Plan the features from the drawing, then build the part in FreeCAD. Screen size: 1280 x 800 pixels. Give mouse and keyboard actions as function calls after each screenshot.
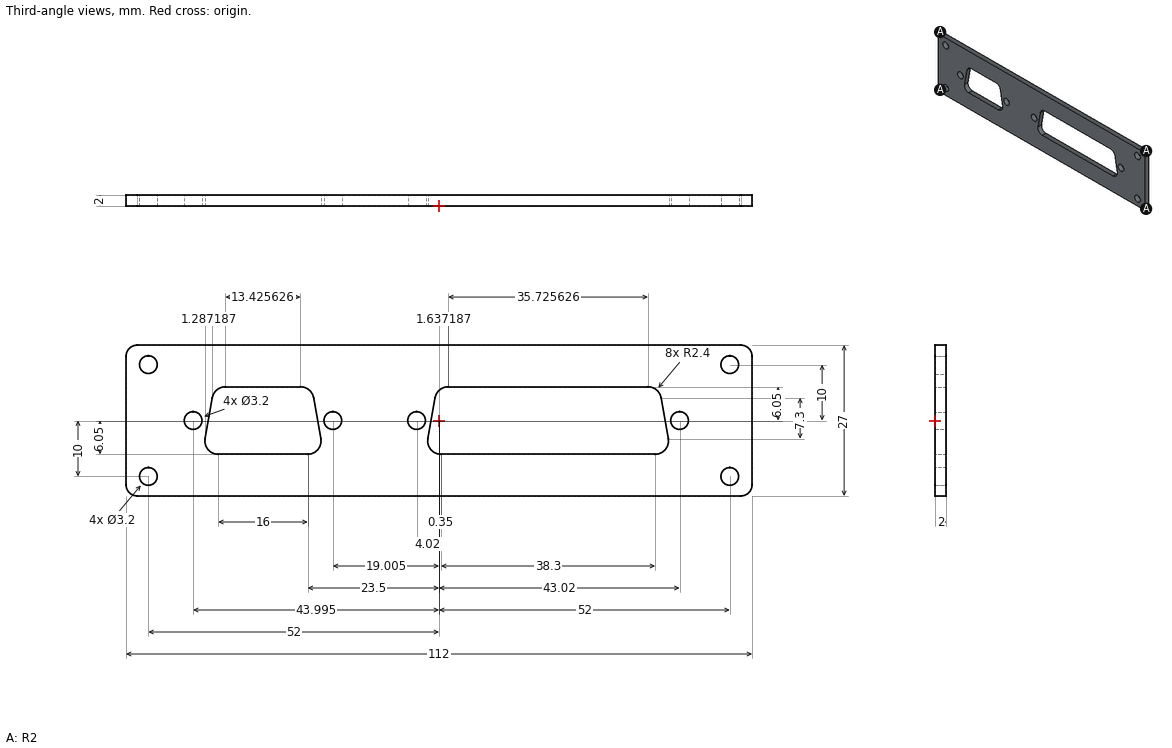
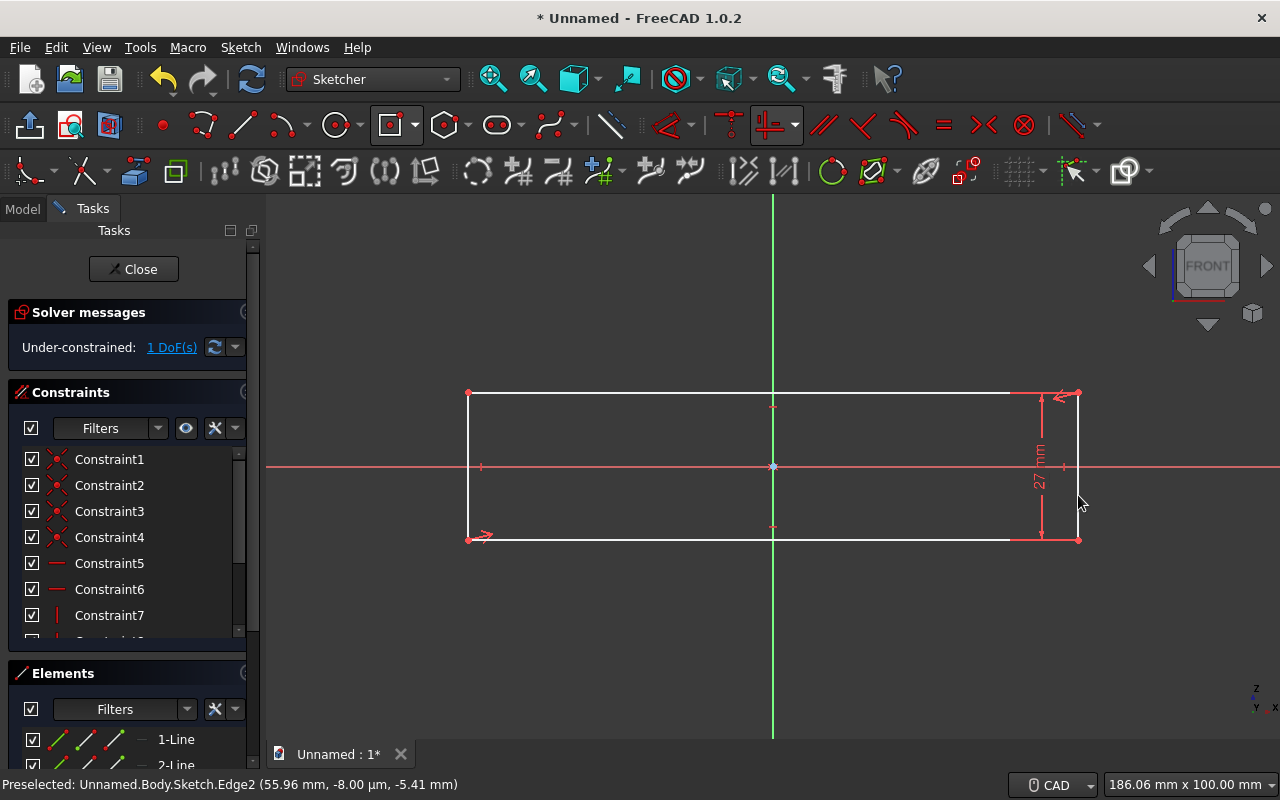
click(651, 540)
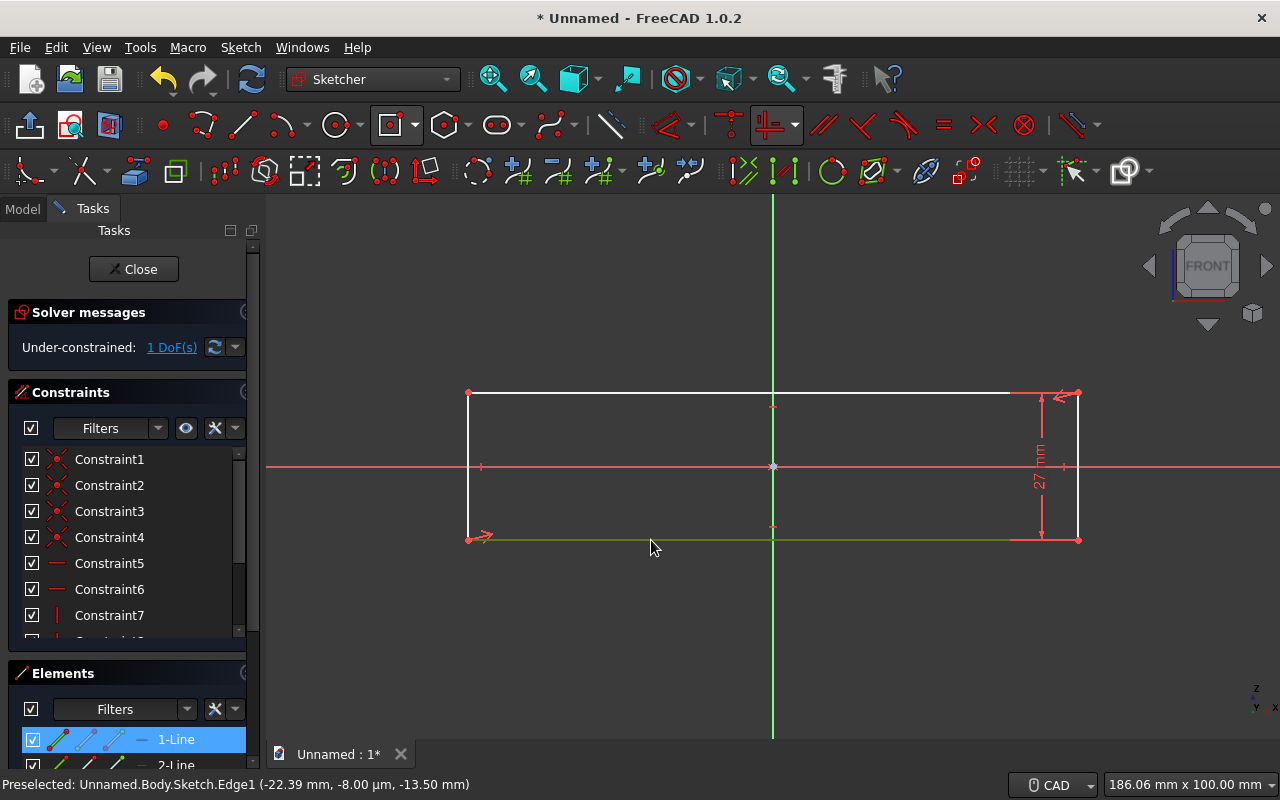
click(694, 126)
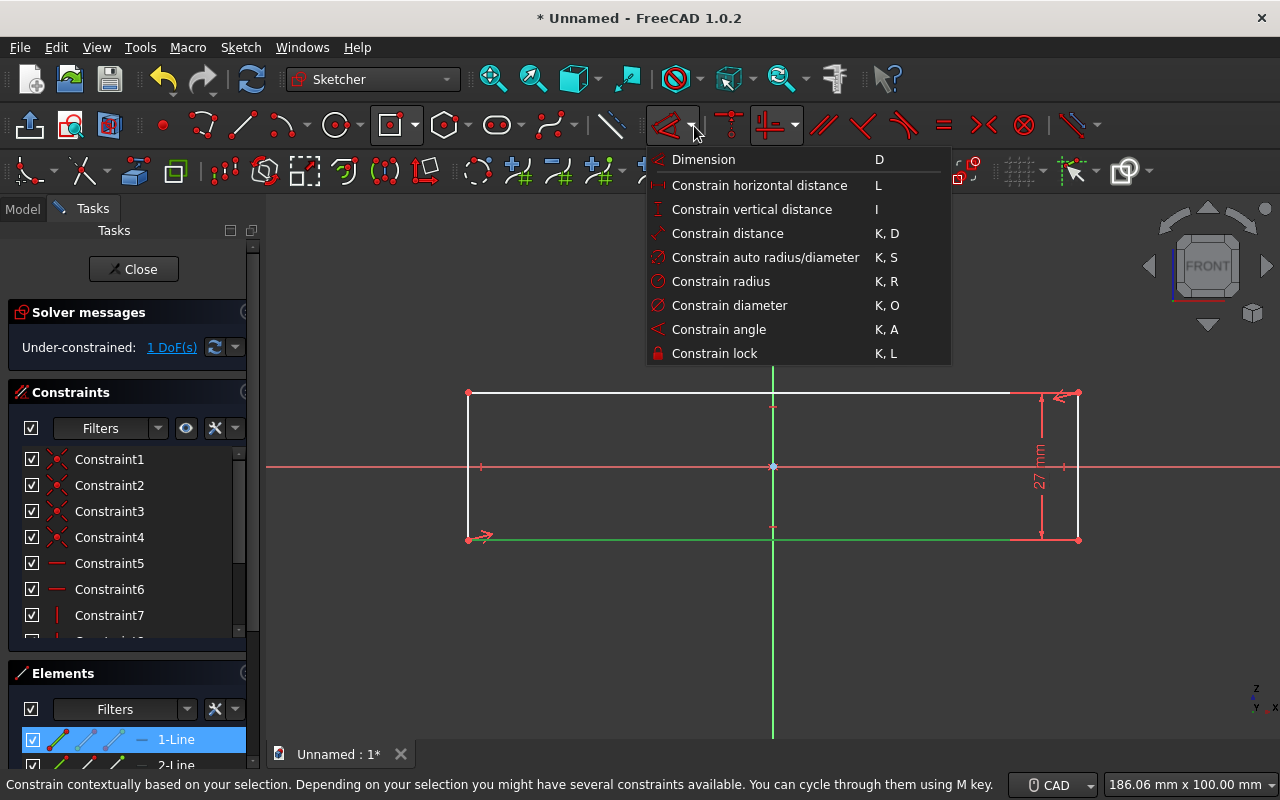
click(799, 185)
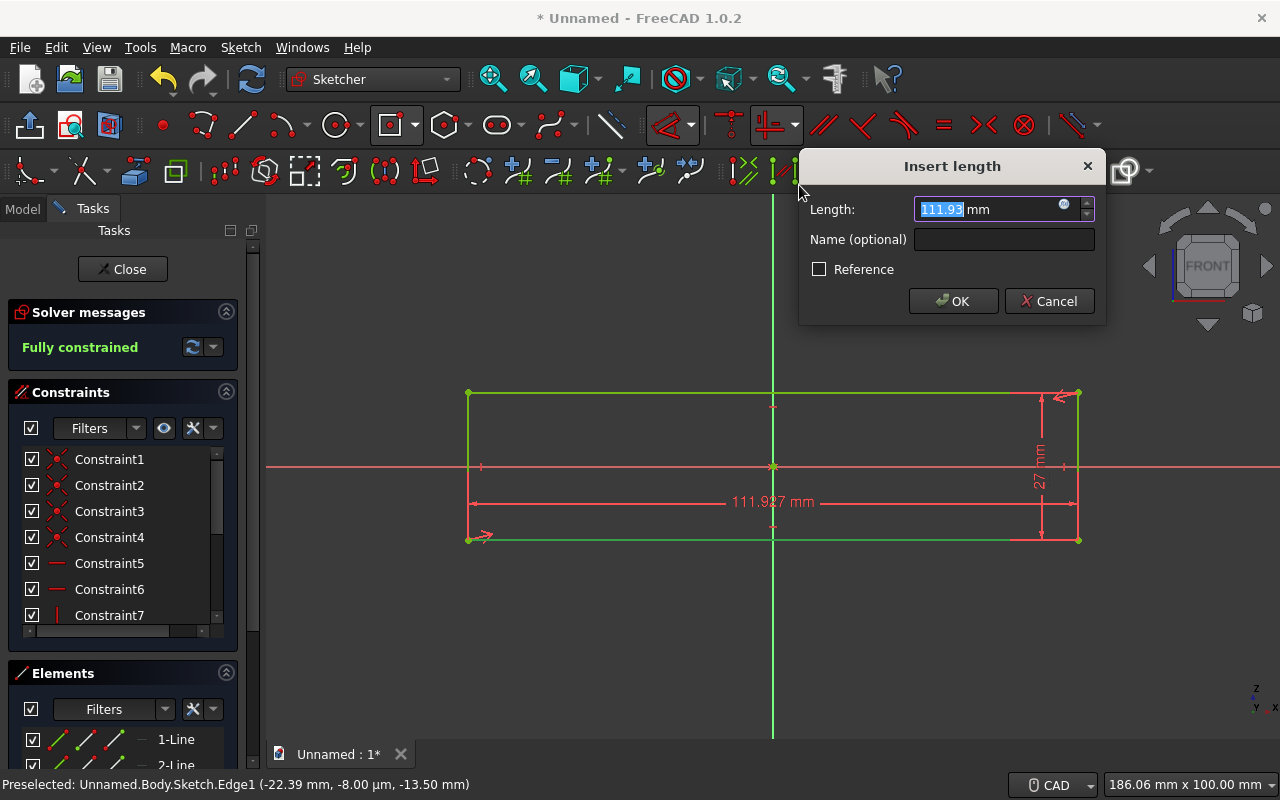
text(112)
key(Return)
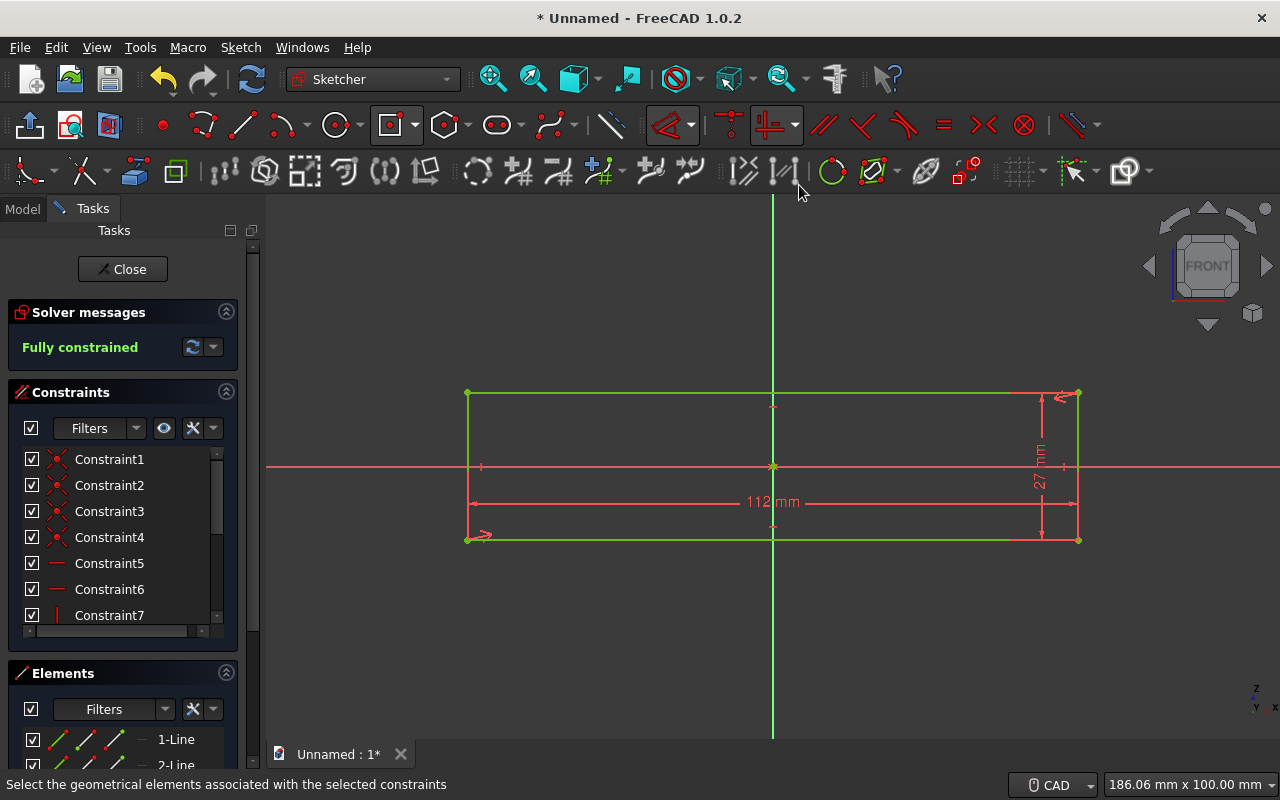
click(123, 269)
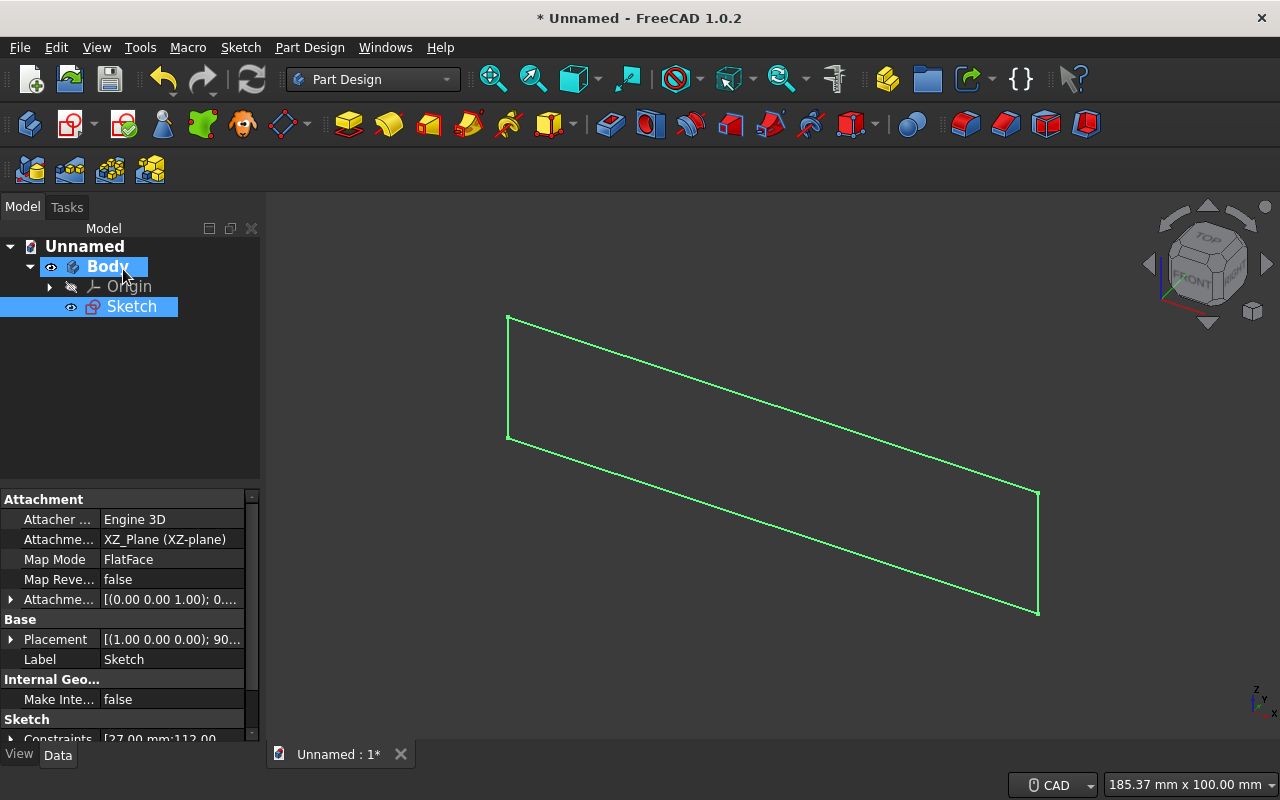
click(350, 124)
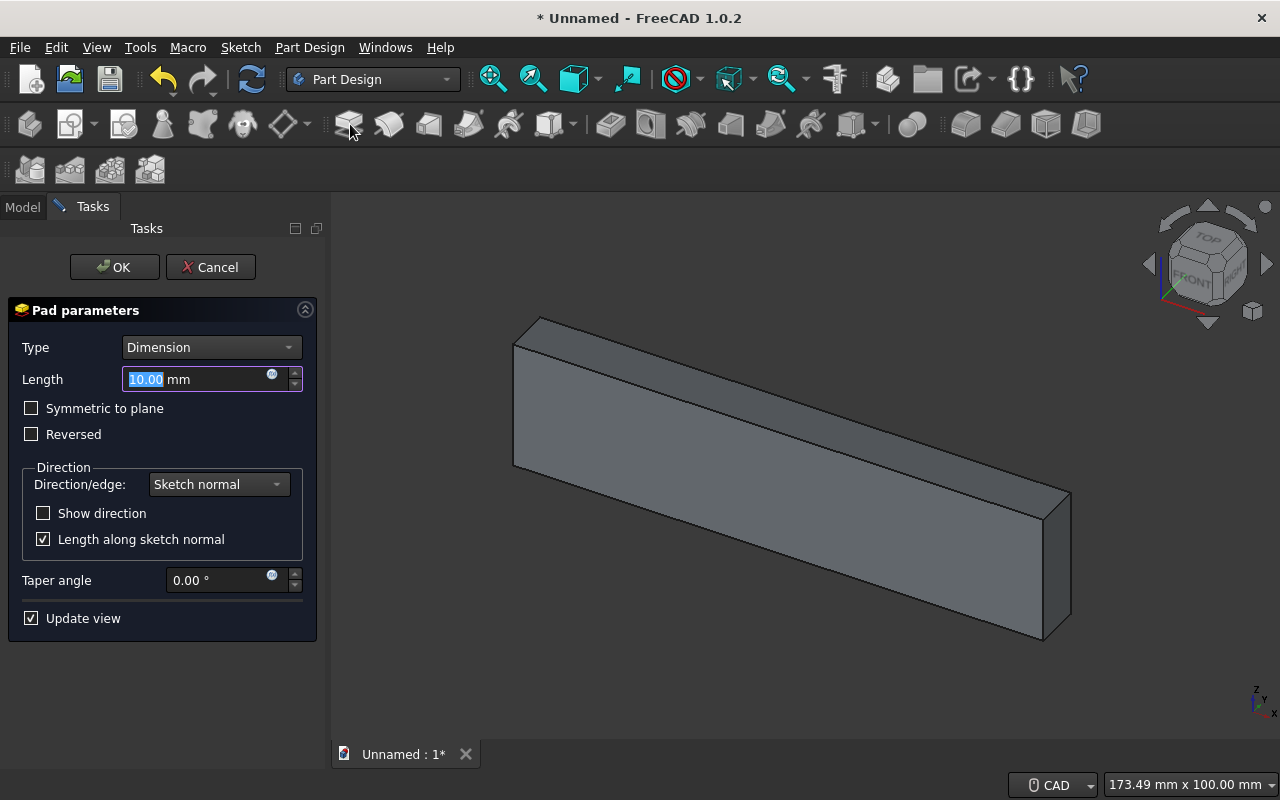
text(2)
key(Tab)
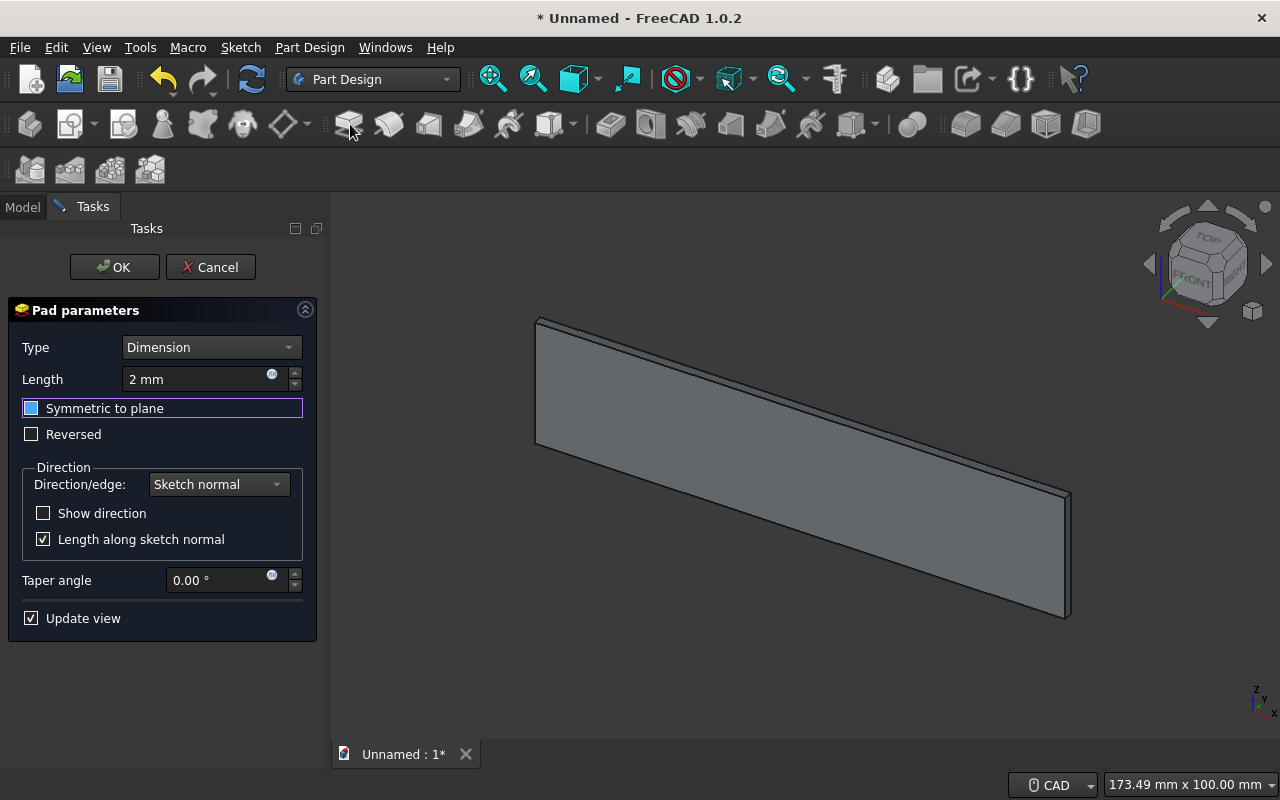
click(30, 434)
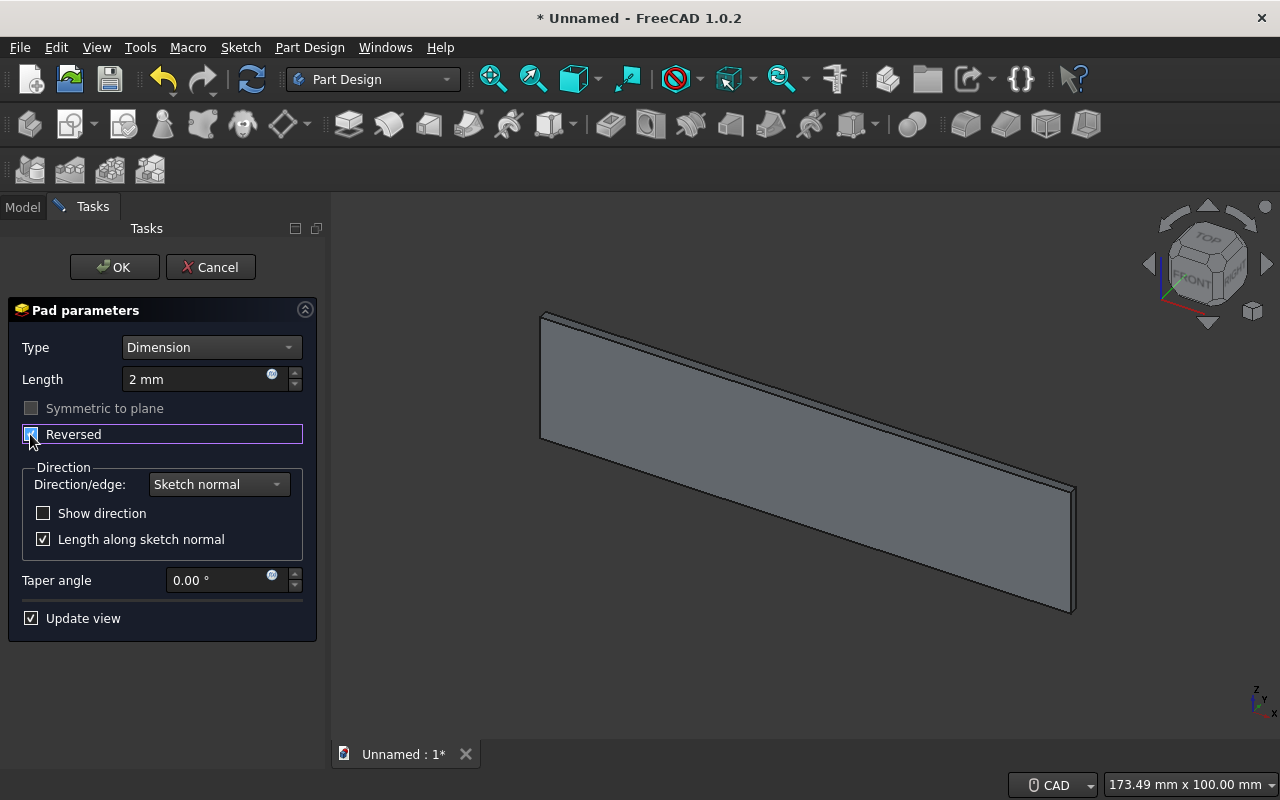
click(115, 267)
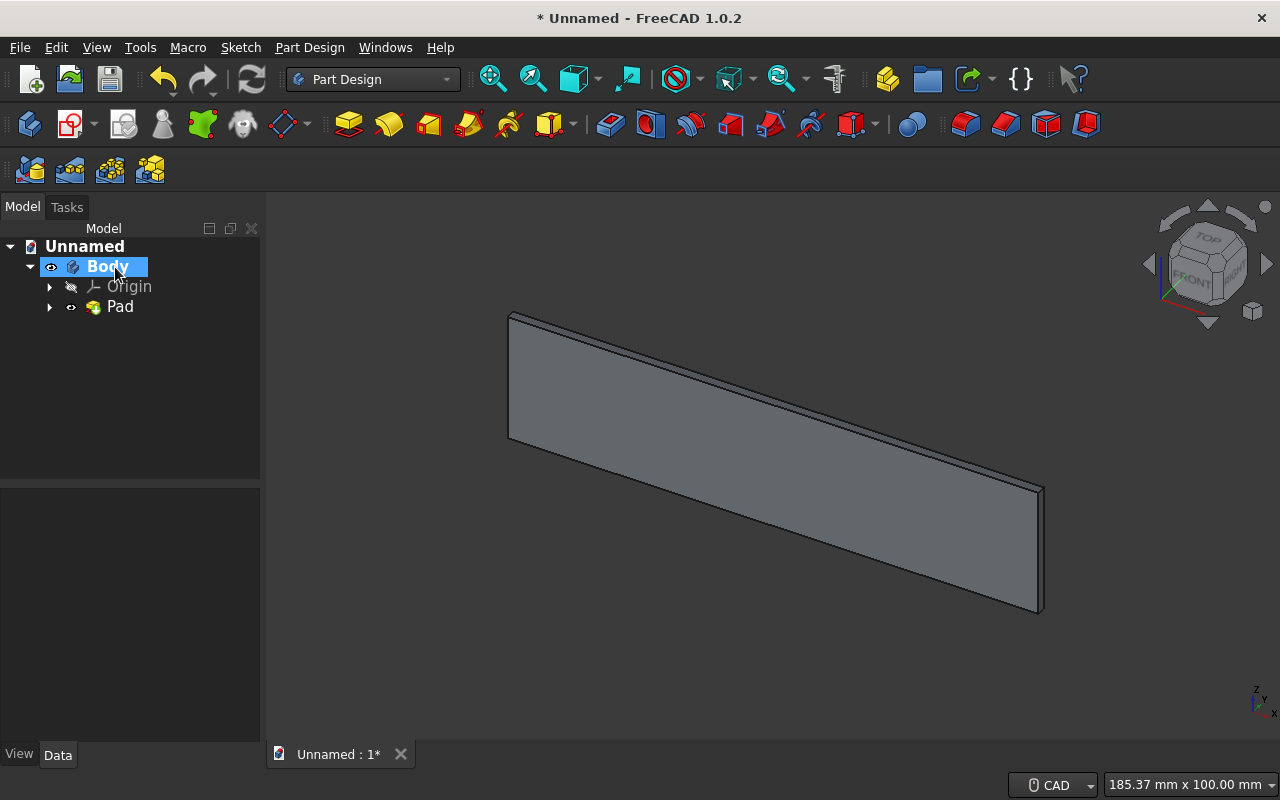
key(4)